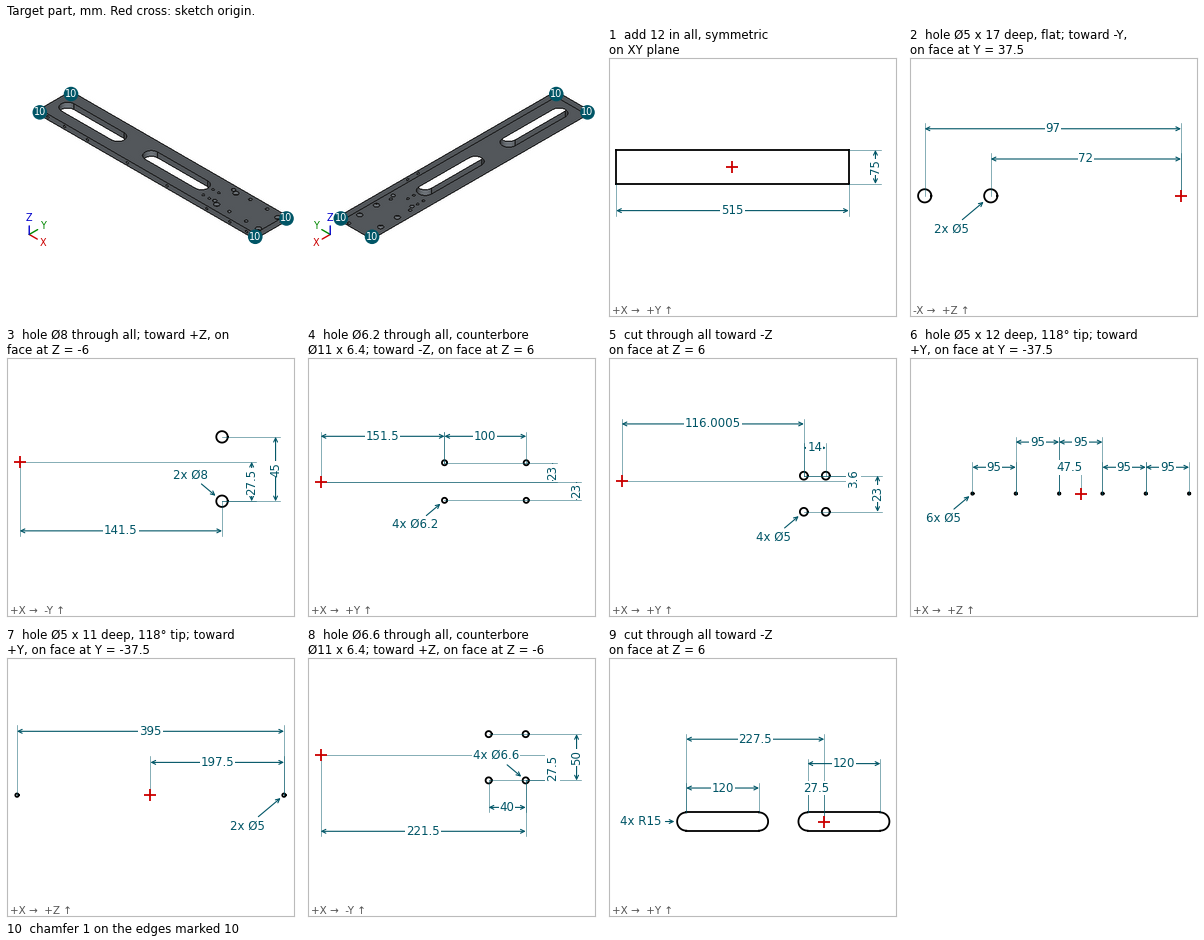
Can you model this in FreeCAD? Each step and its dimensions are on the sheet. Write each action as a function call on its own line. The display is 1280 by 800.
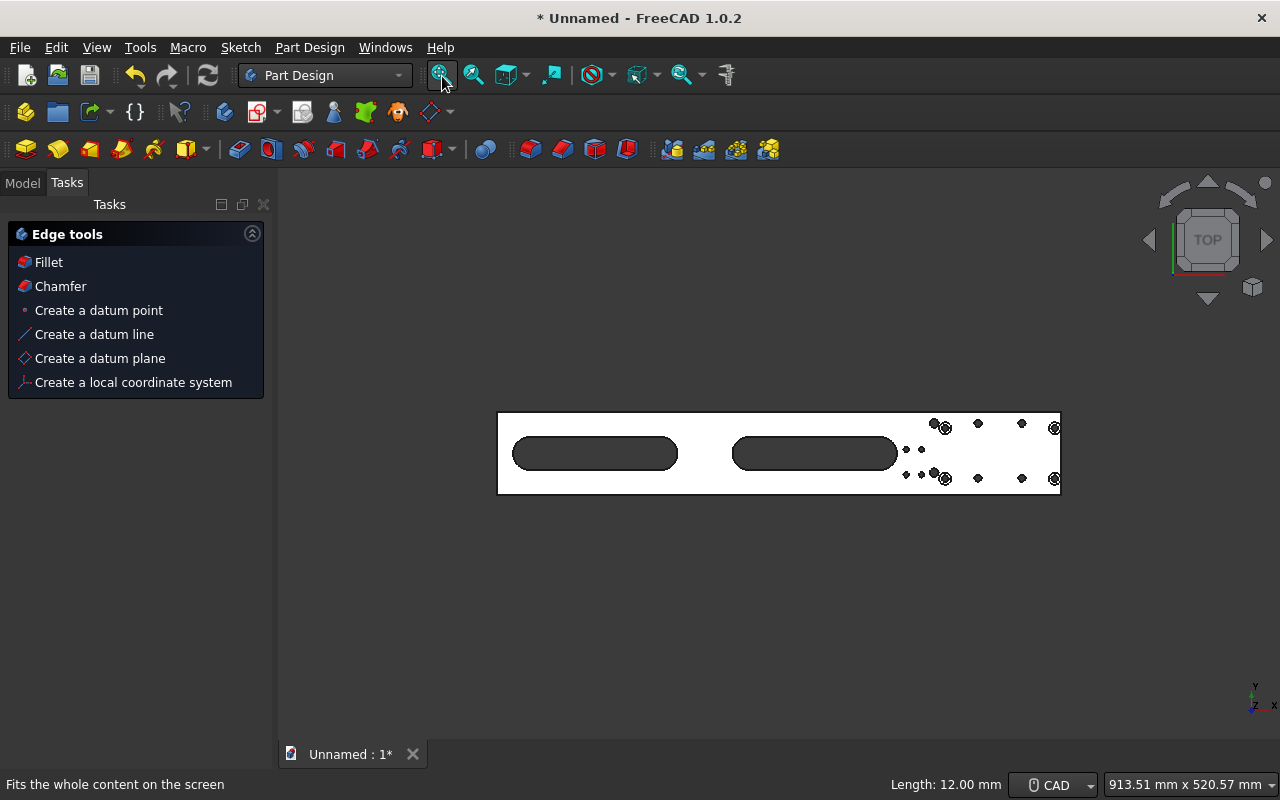
key(0)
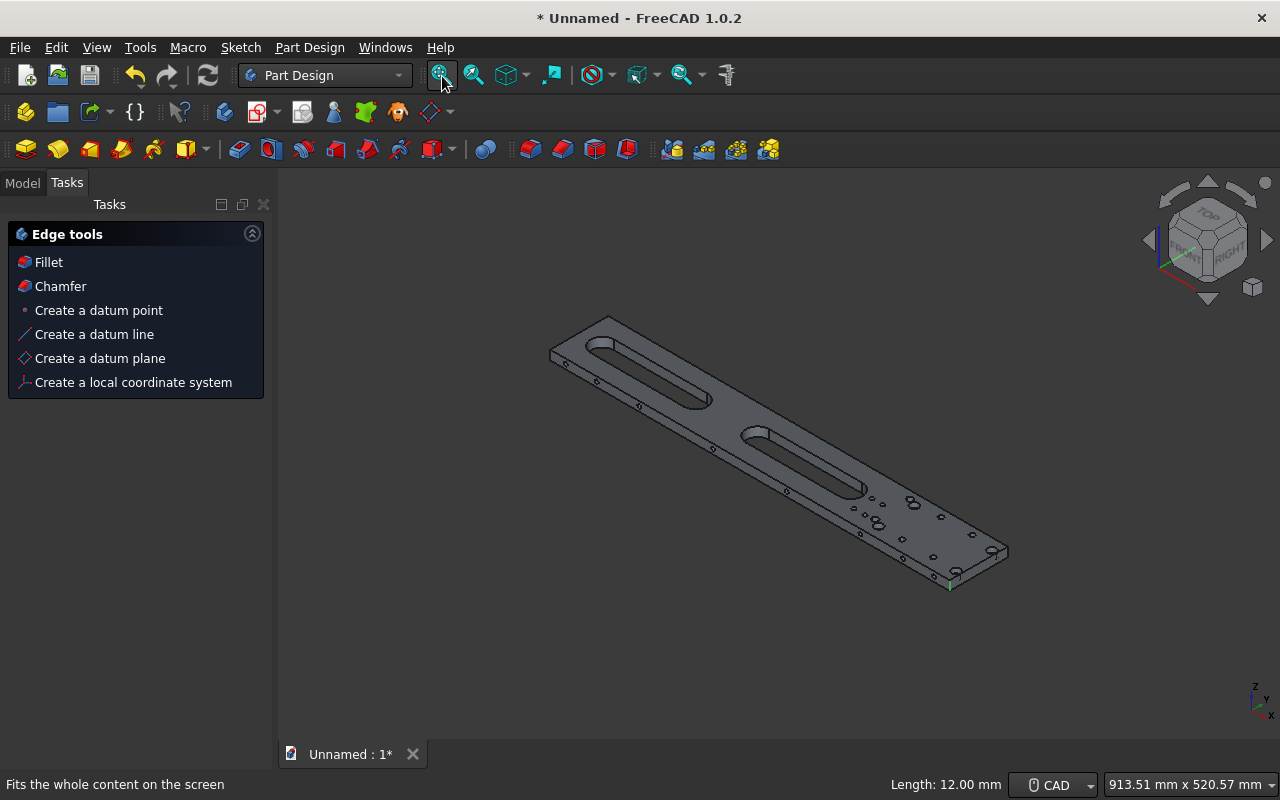
scroll(550, 354, up, 6)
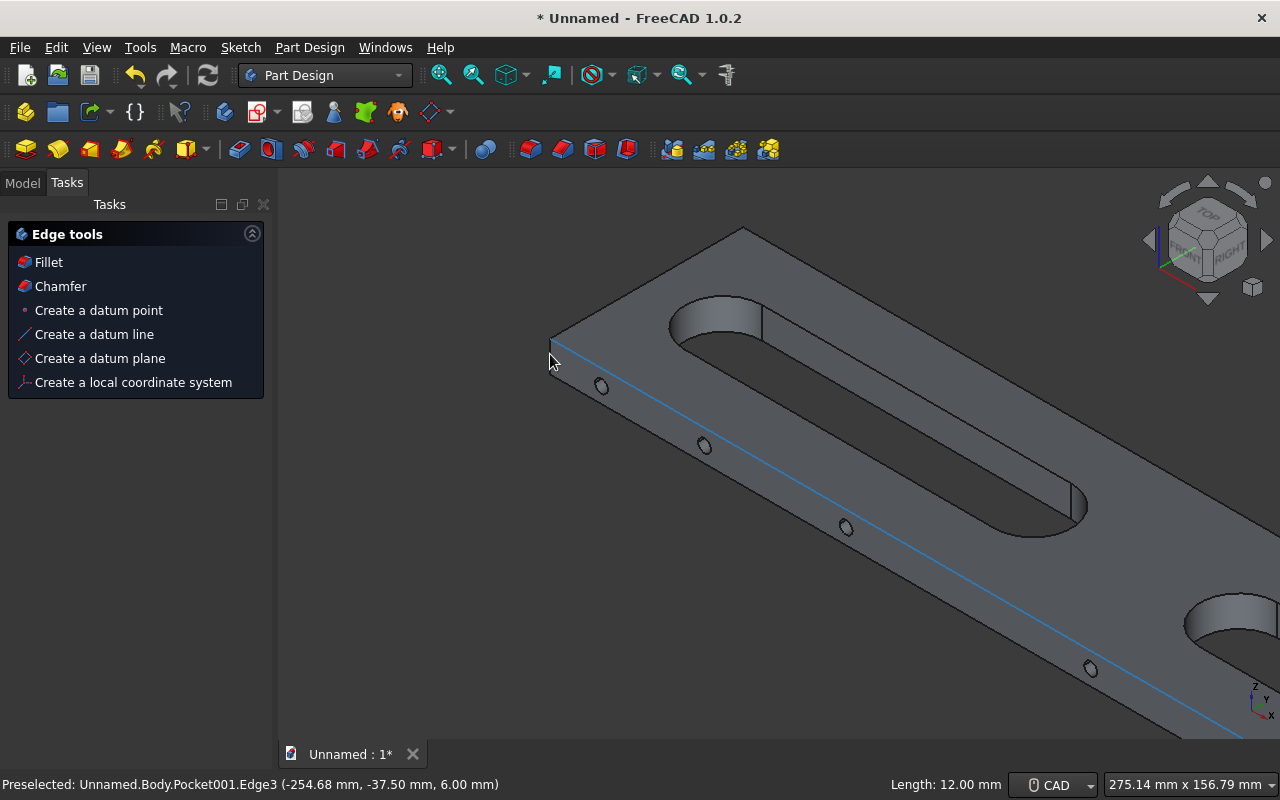
key(v)
key(f)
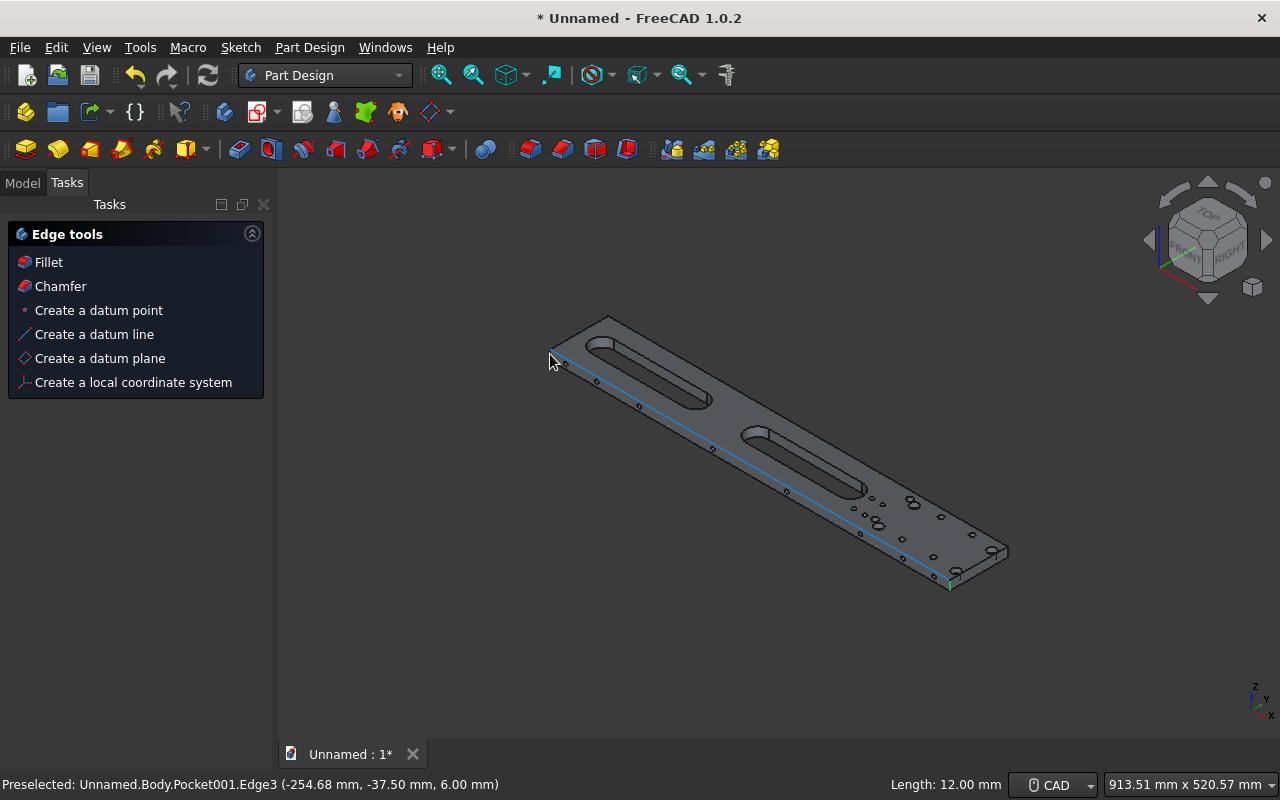
key(1)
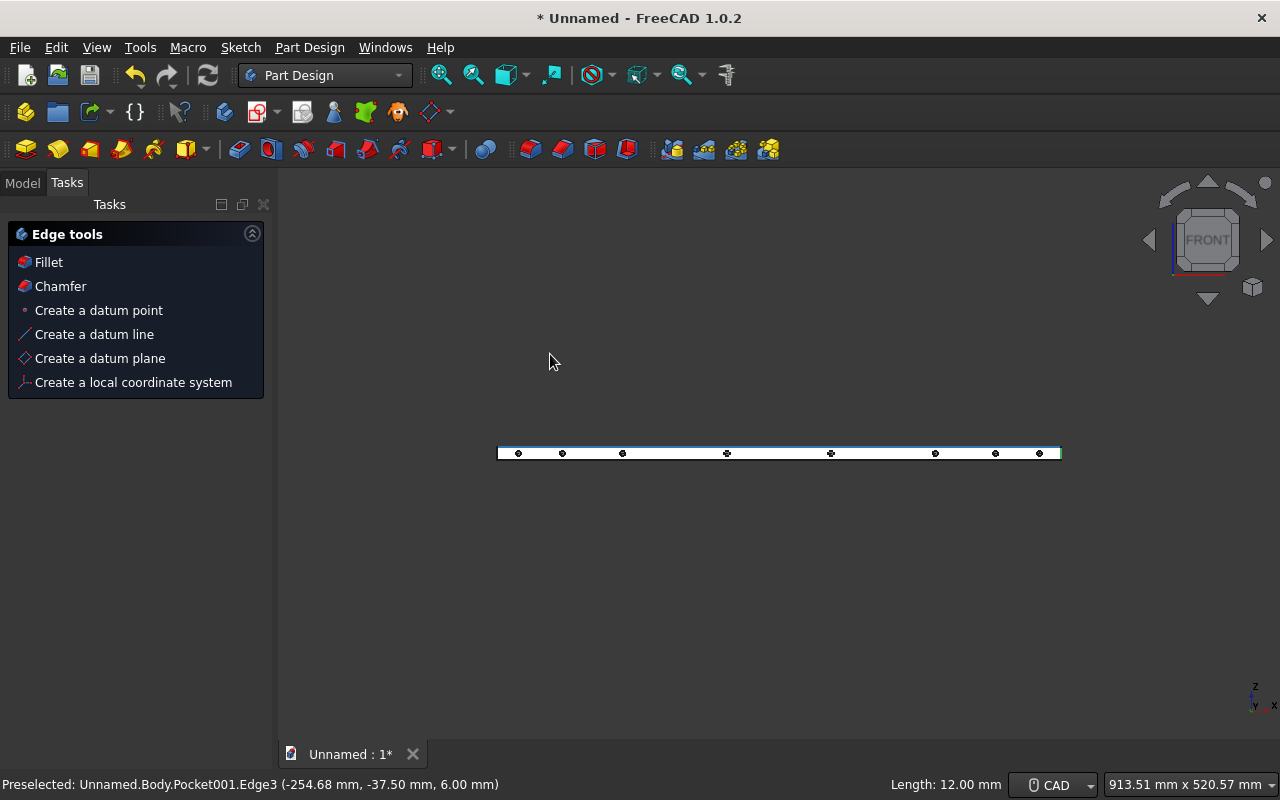
click(497, 452, ctrl)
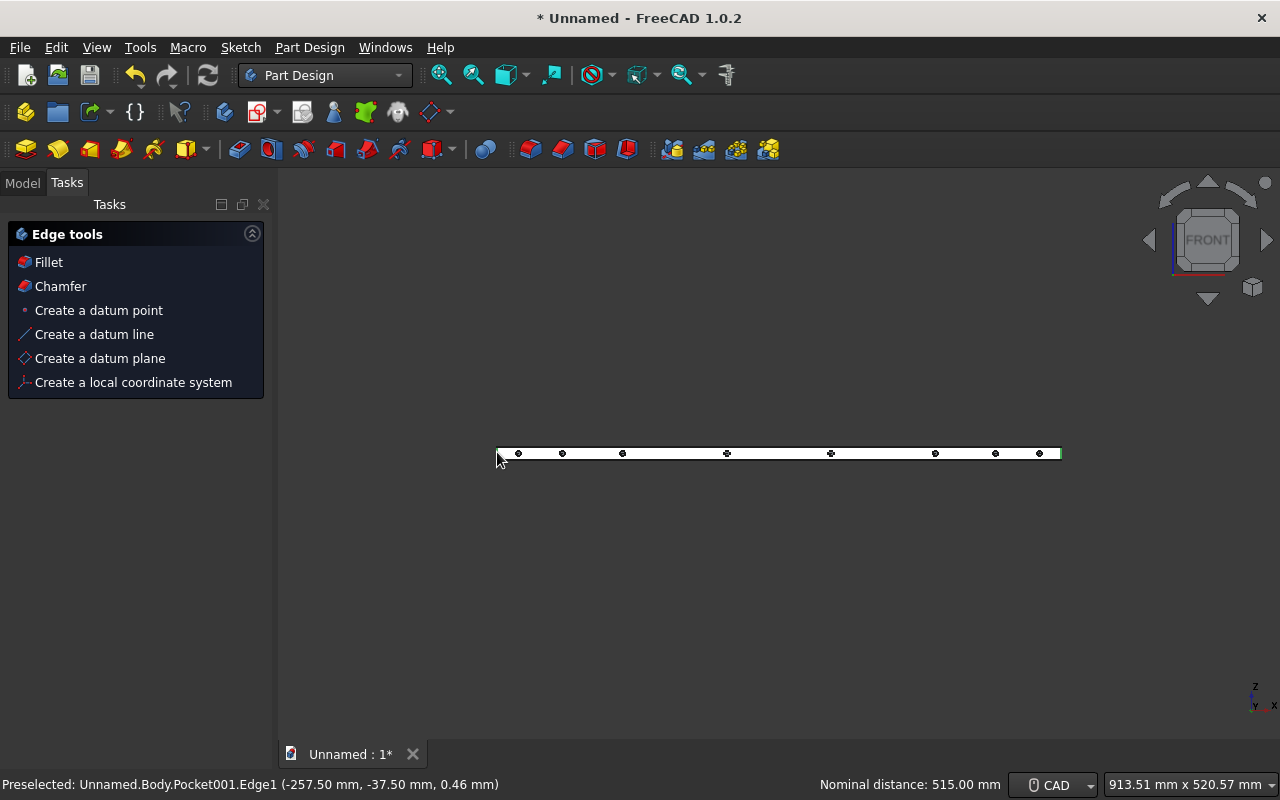
scroll(497, 452, up, 6)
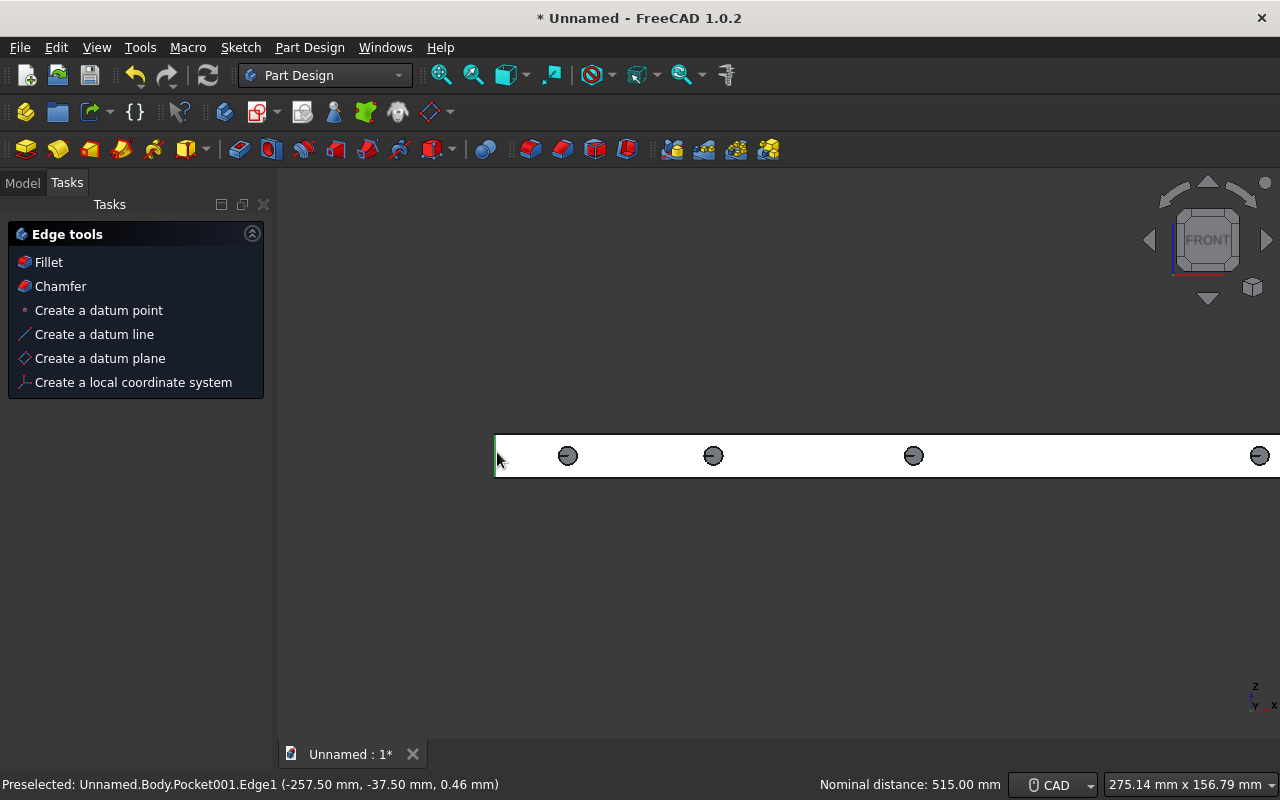
key(v)
key(f)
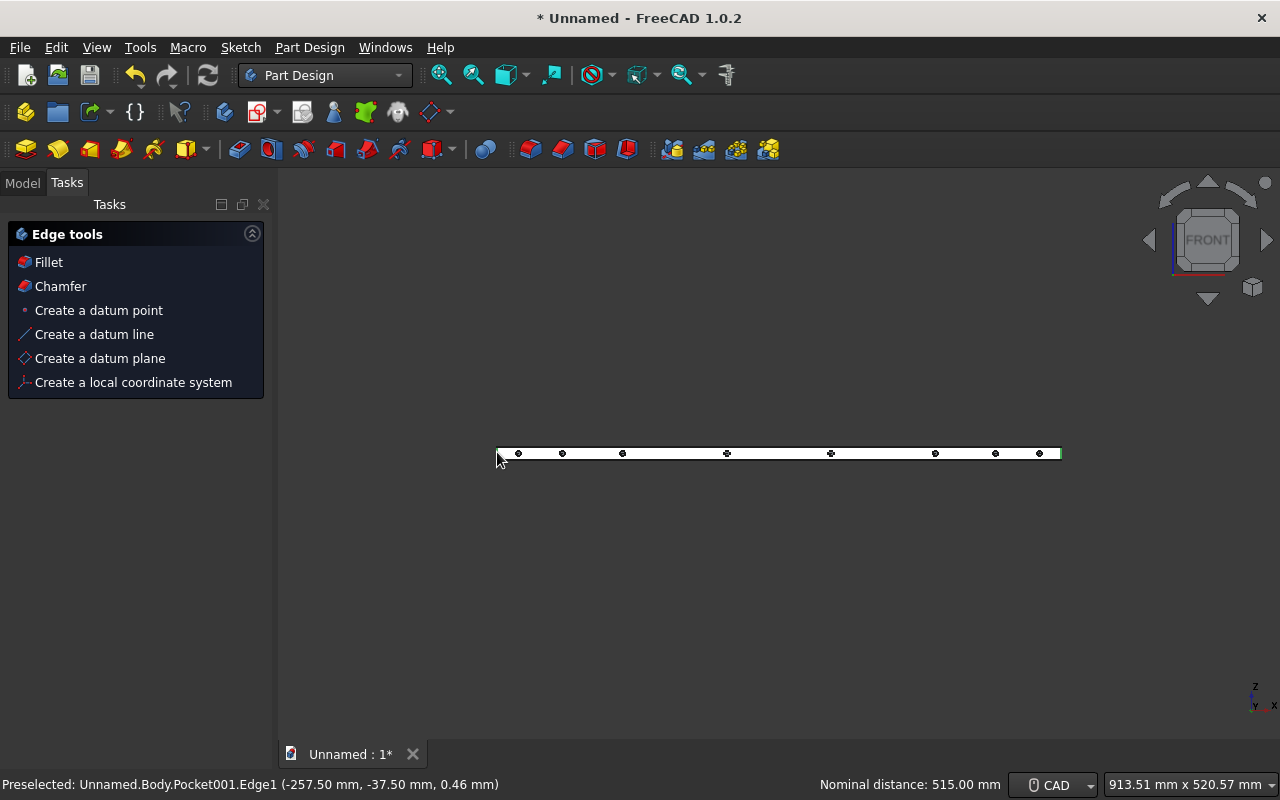
key(3)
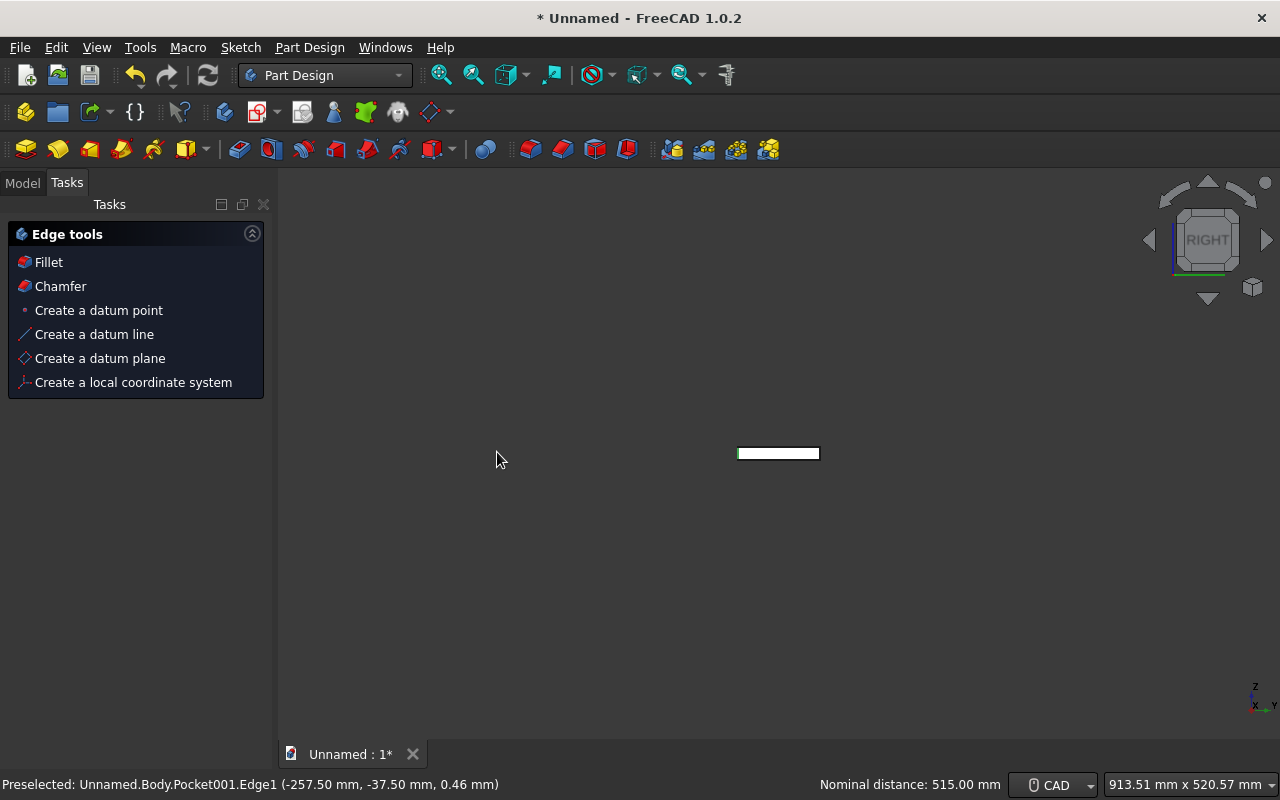
key(v)
key(f)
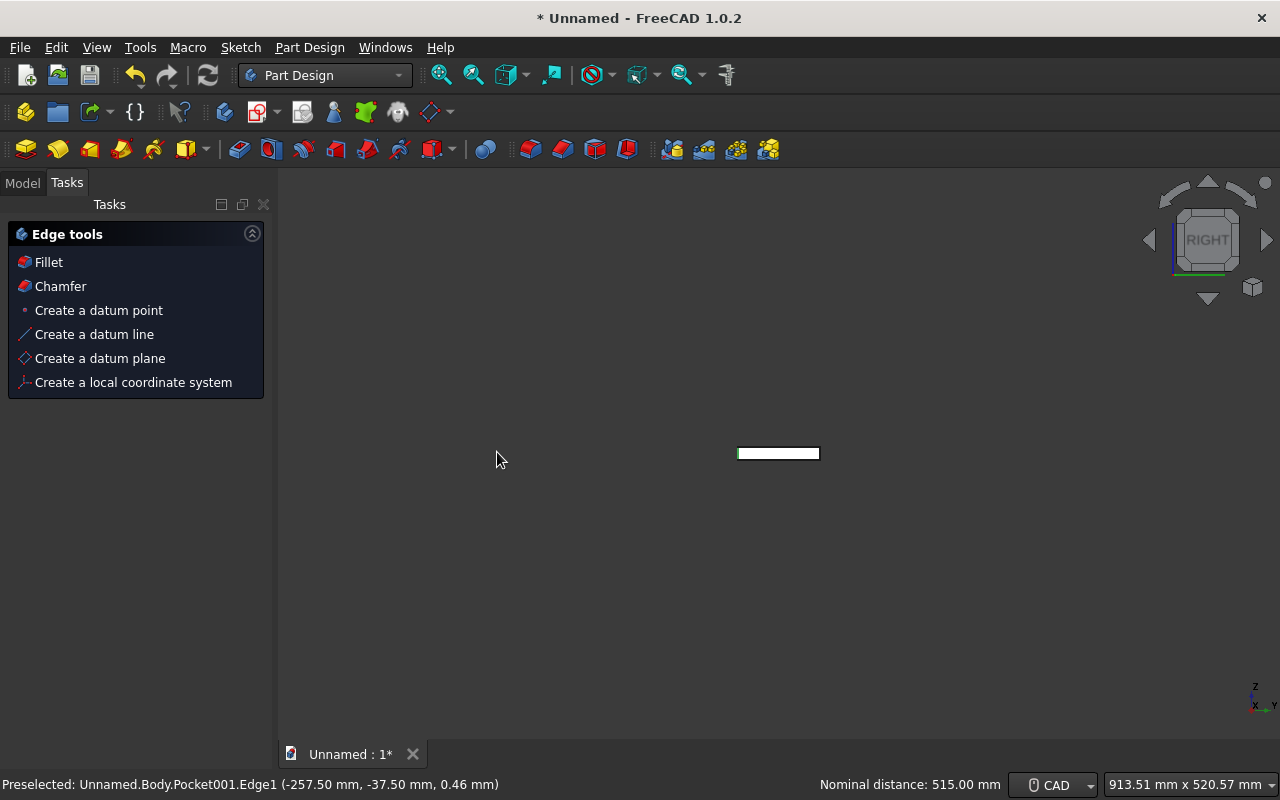
click(820, 452, ctrl)